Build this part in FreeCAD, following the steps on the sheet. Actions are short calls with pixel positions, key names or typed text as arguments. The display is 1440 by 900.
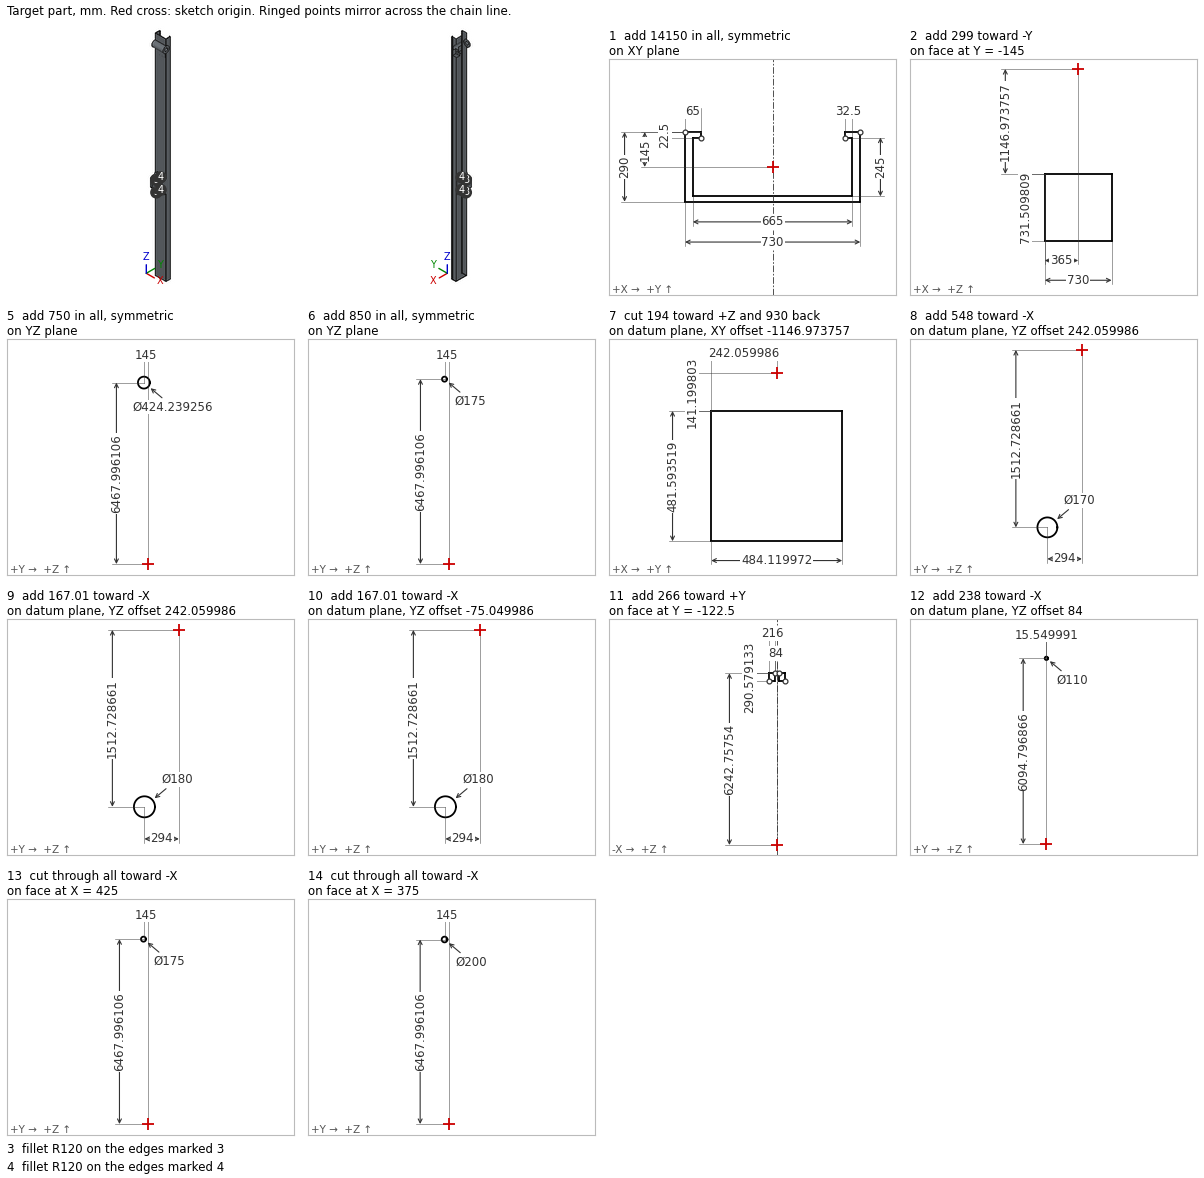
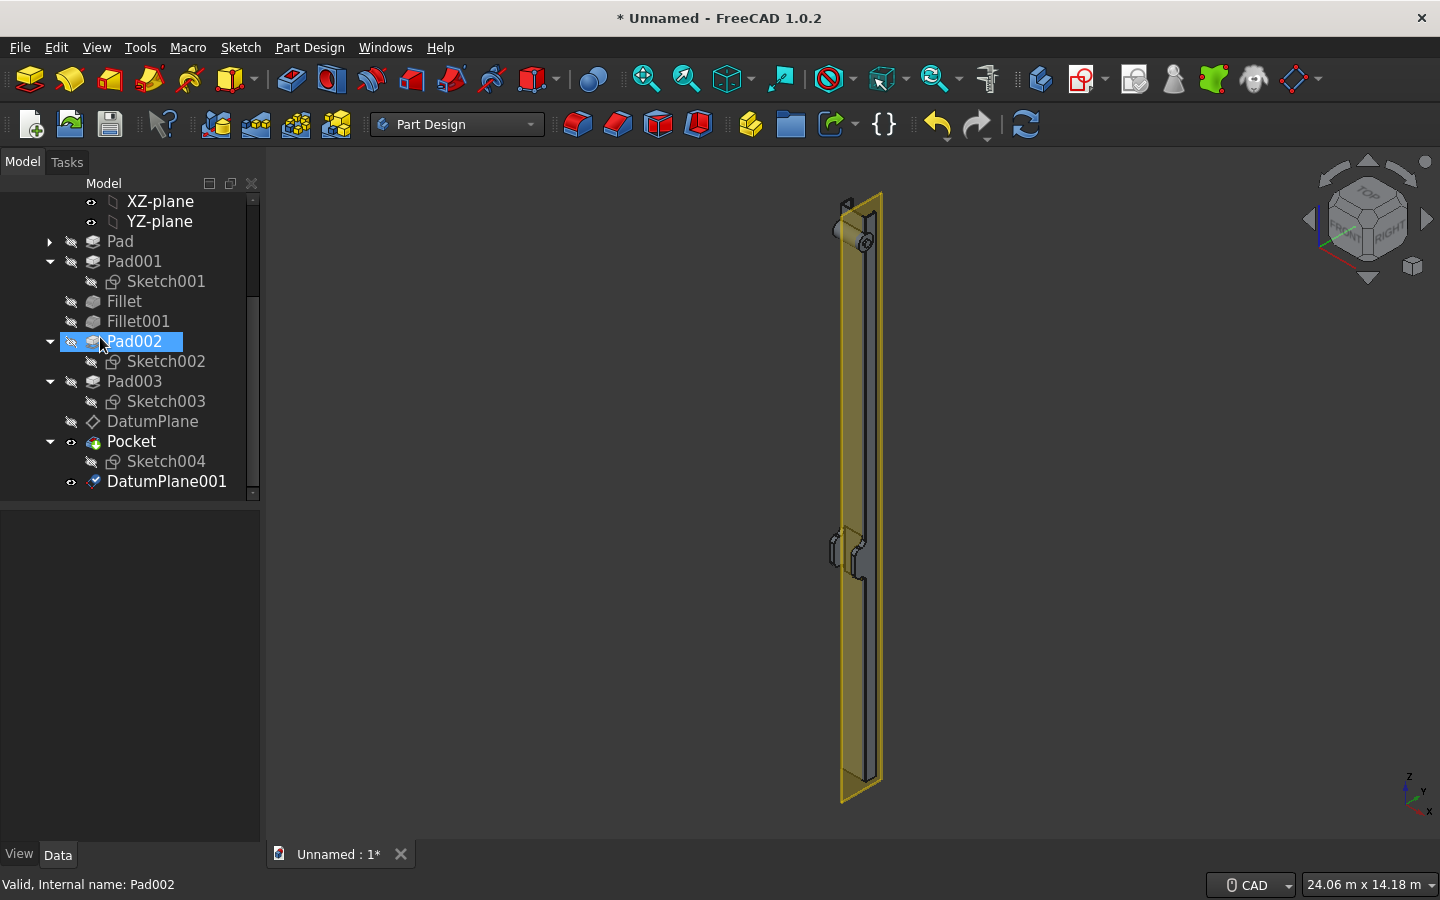
click(116, 482)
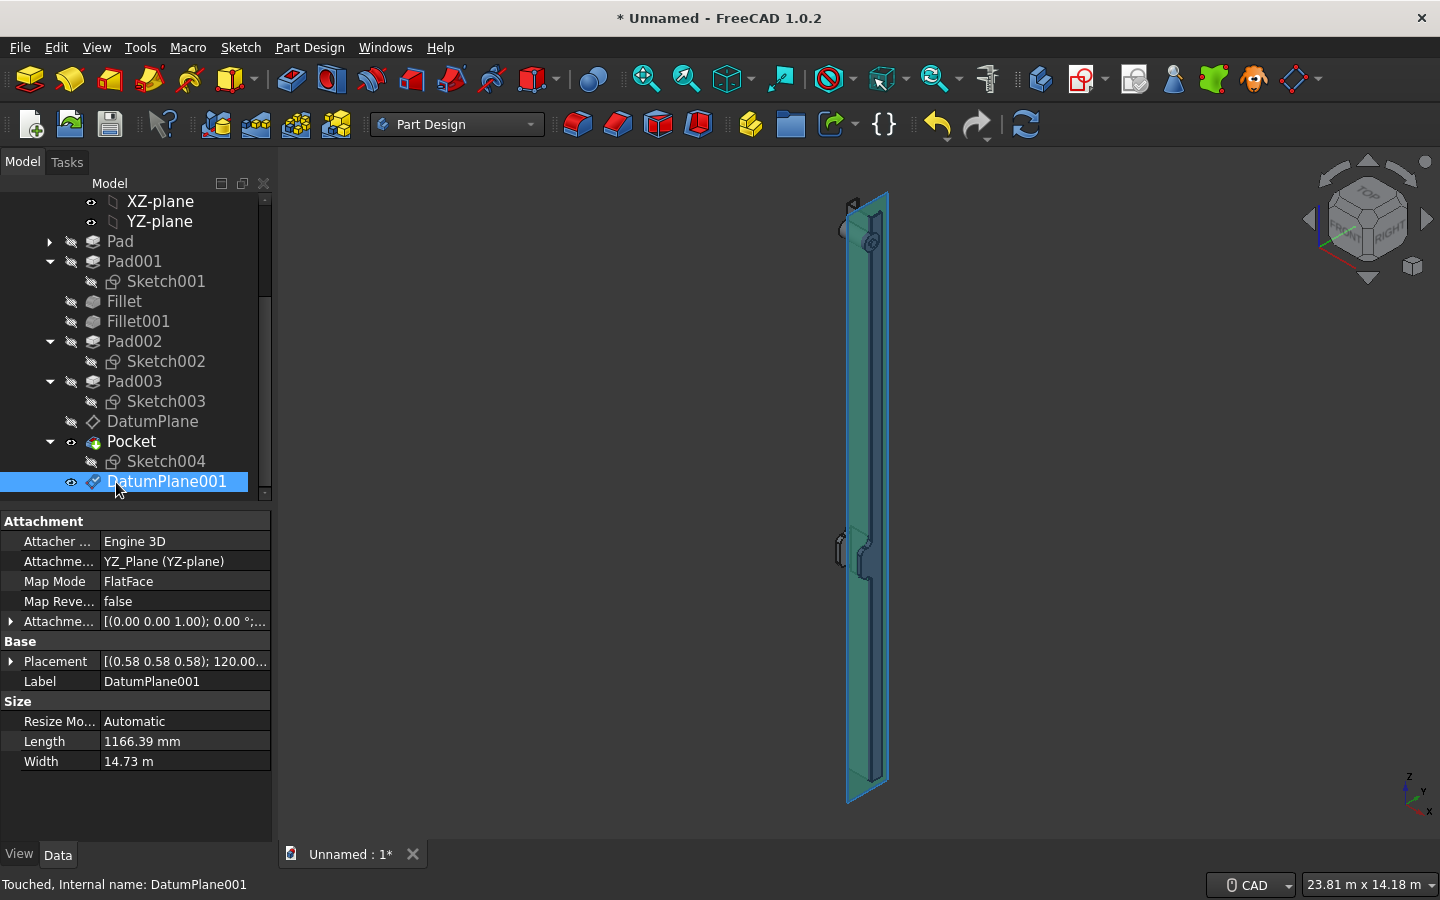
click(1082, 80)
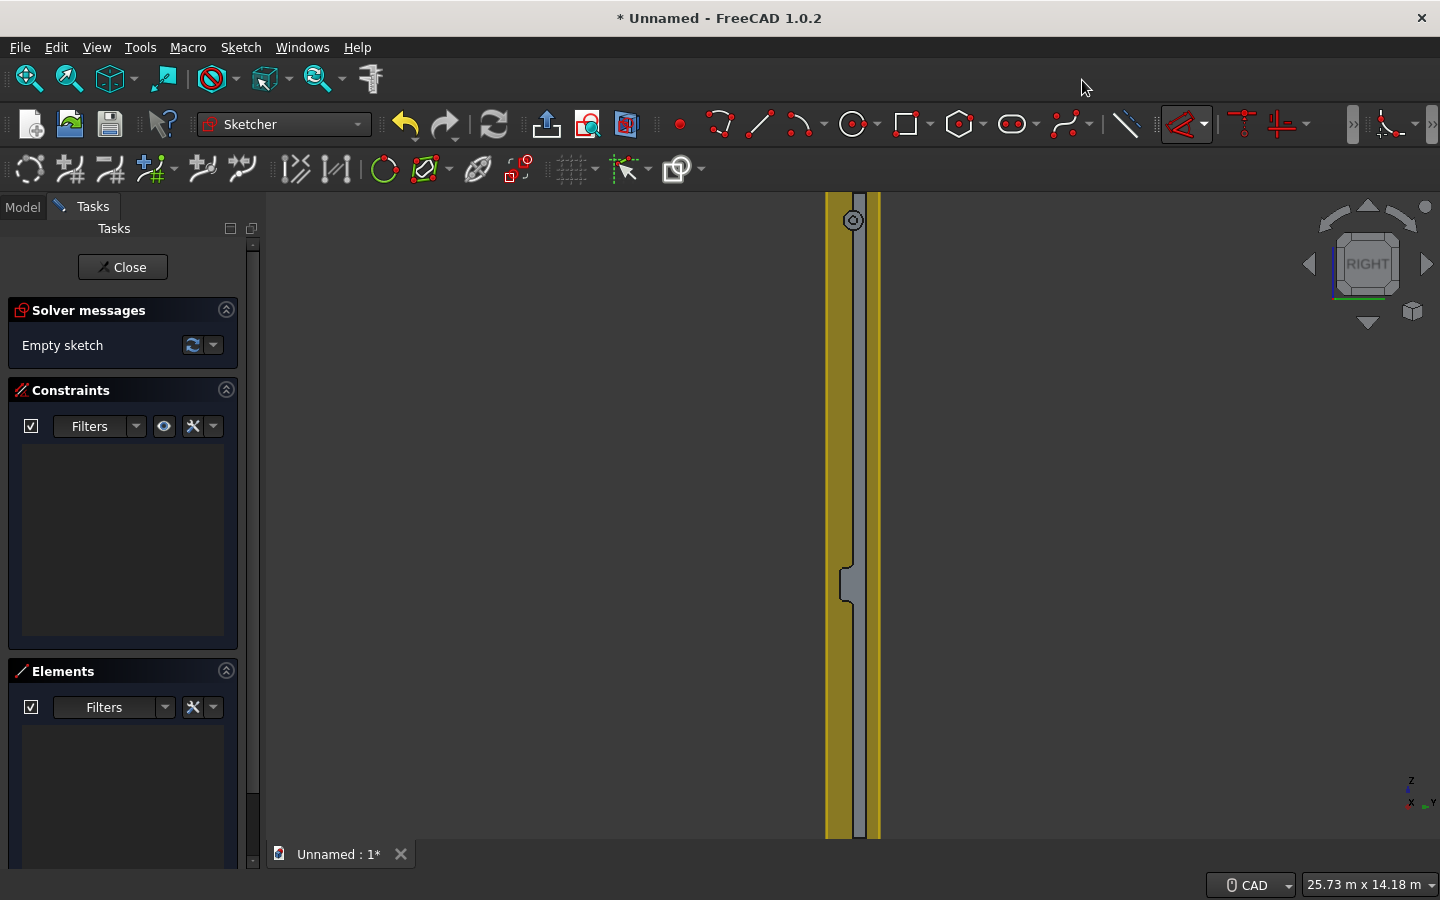
key(q)
key(s)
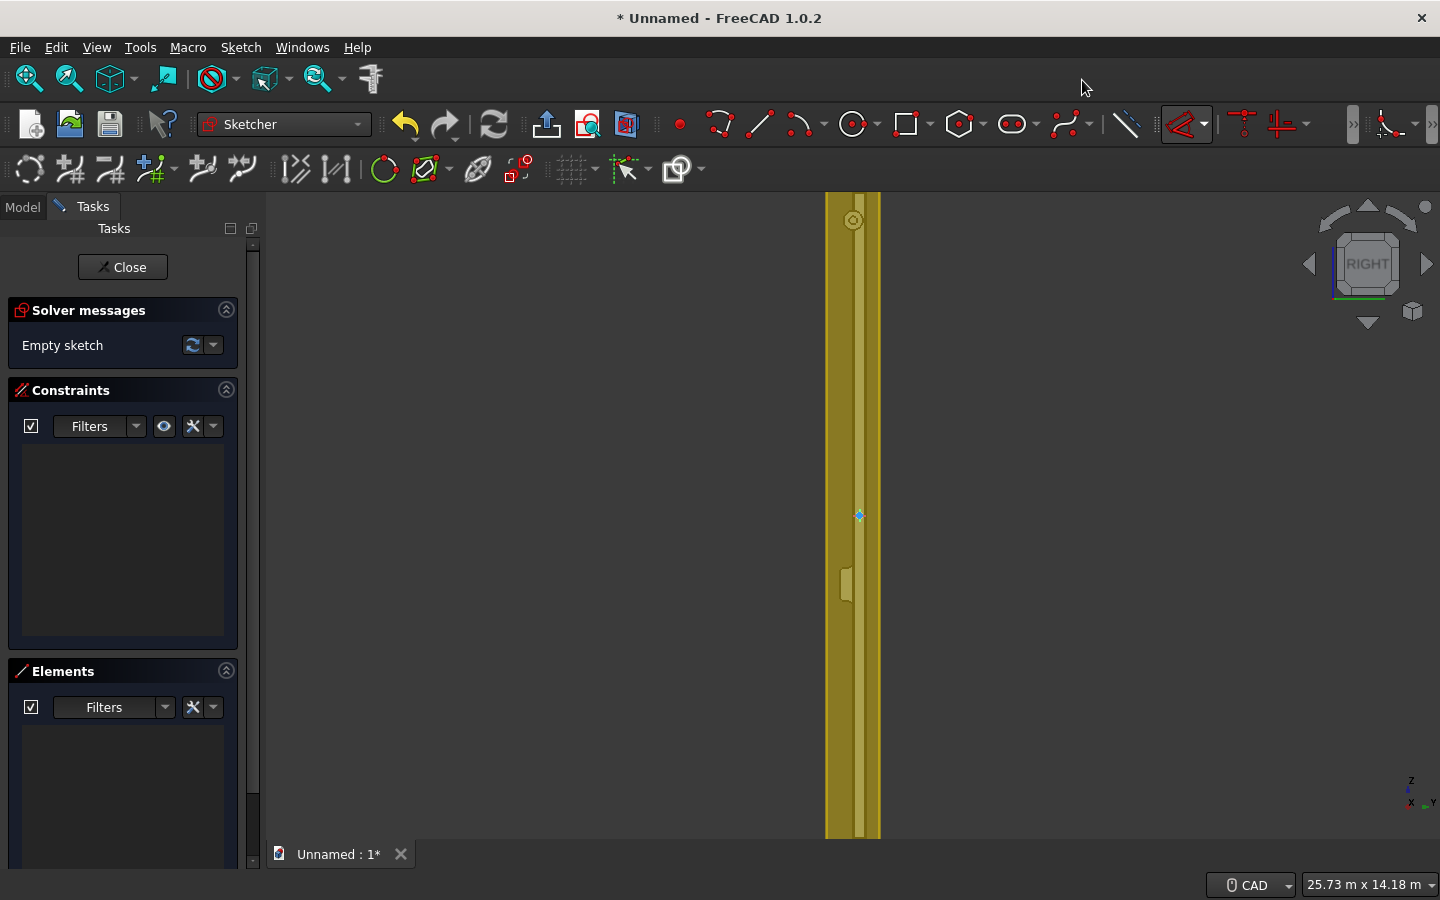
scroll(850, 588, up, 15)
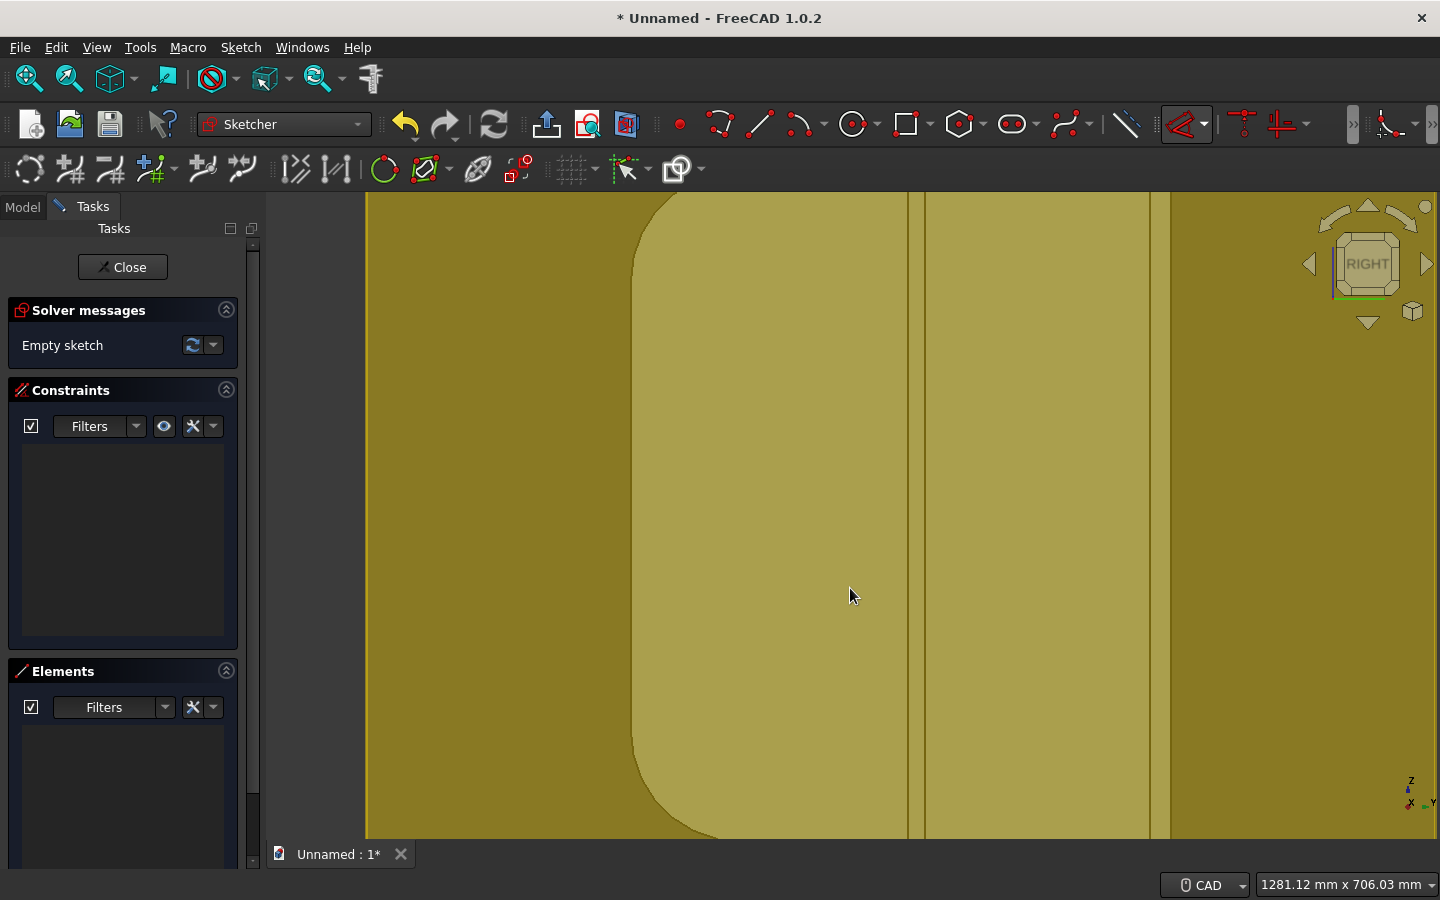
scroll(759, 501, up, 5)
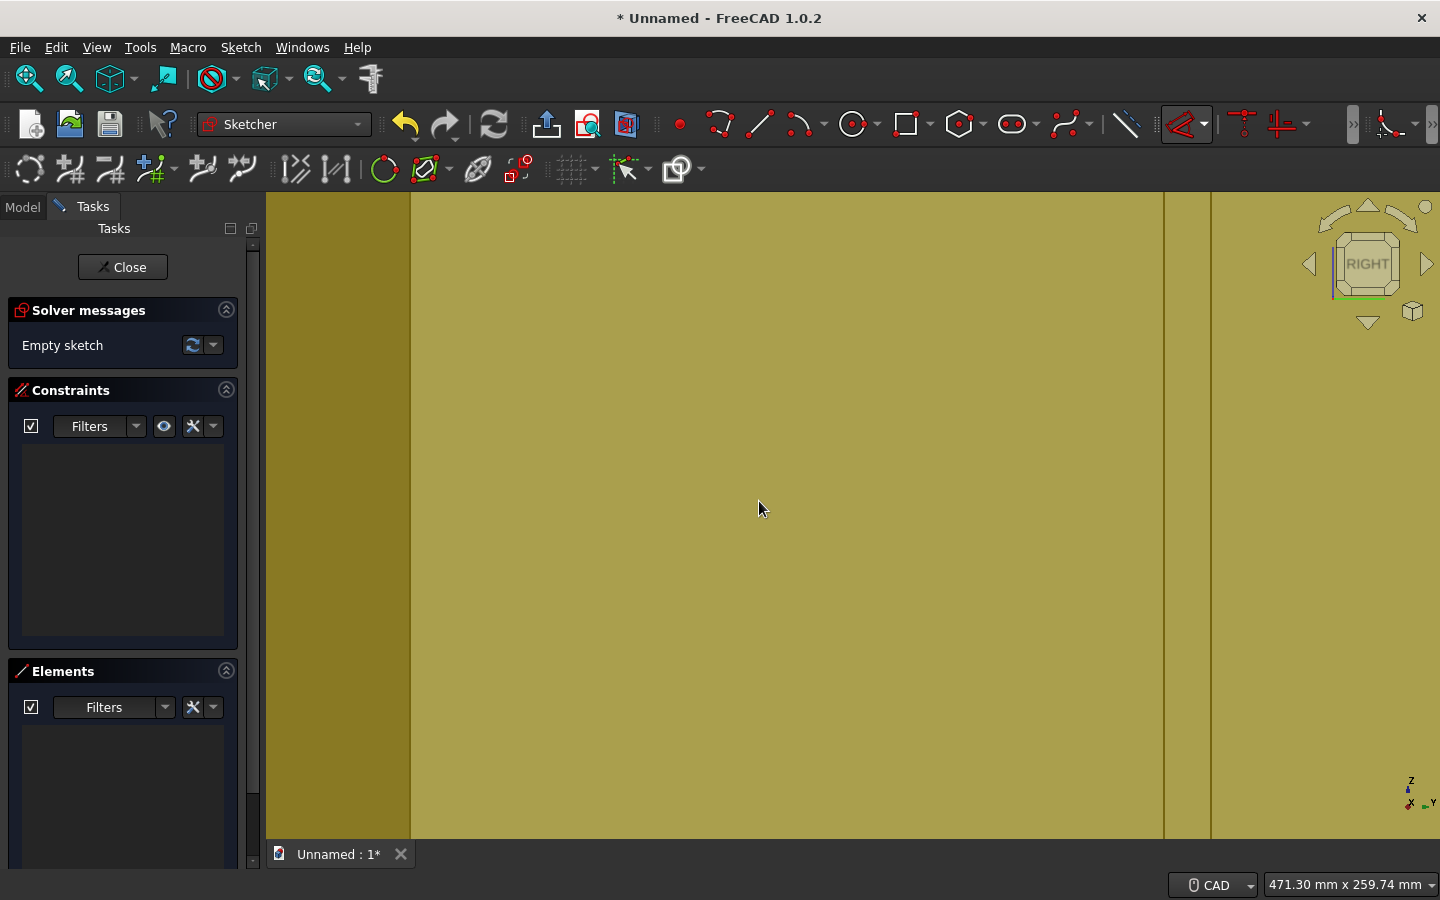
key(g)
key(c)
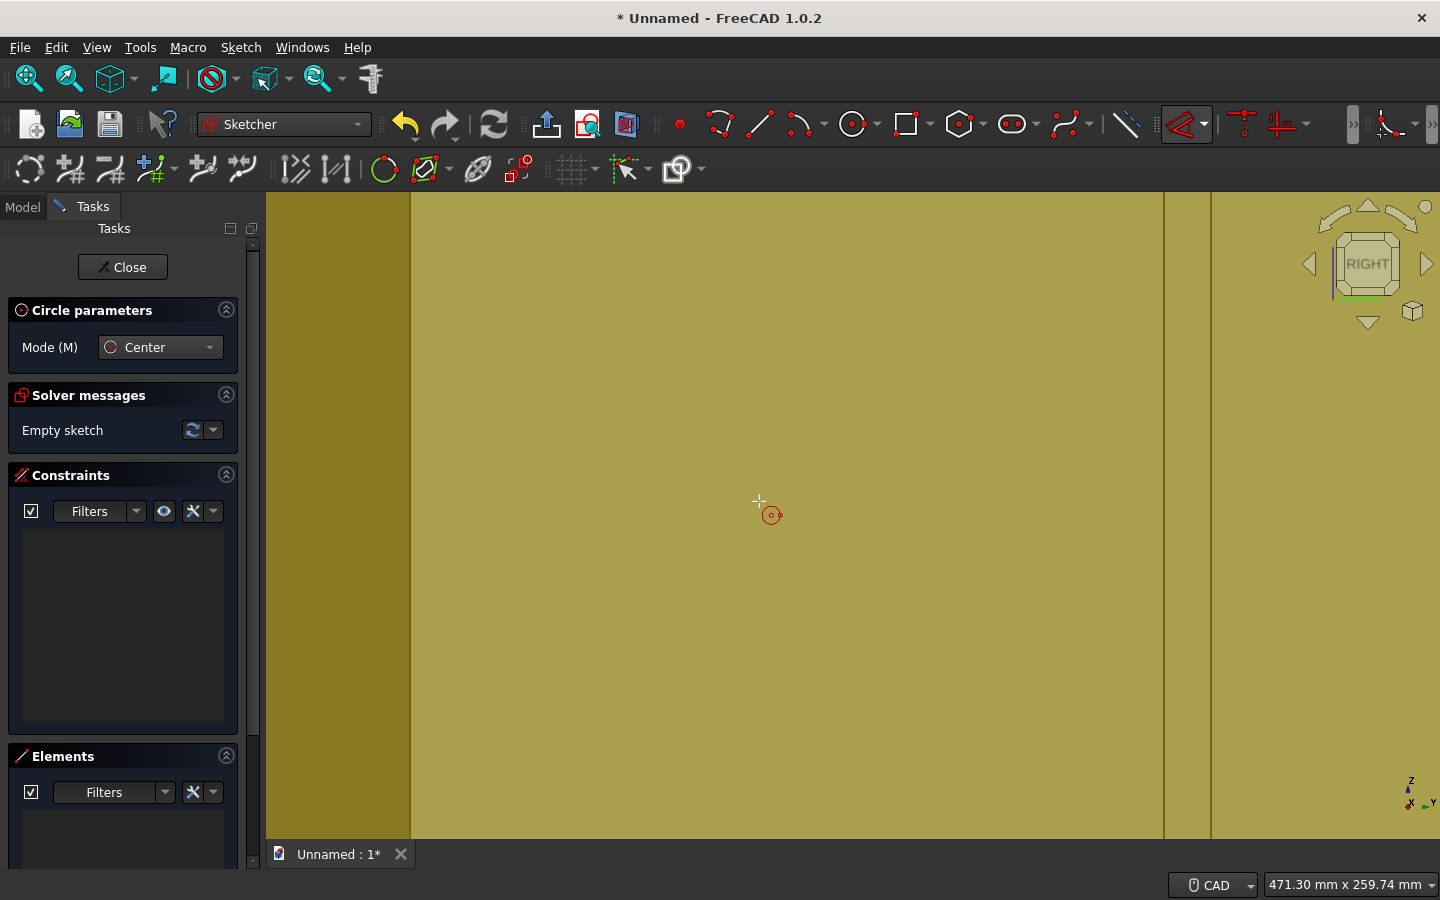
click(784, 515)
click(933, 365)
key(Escape)